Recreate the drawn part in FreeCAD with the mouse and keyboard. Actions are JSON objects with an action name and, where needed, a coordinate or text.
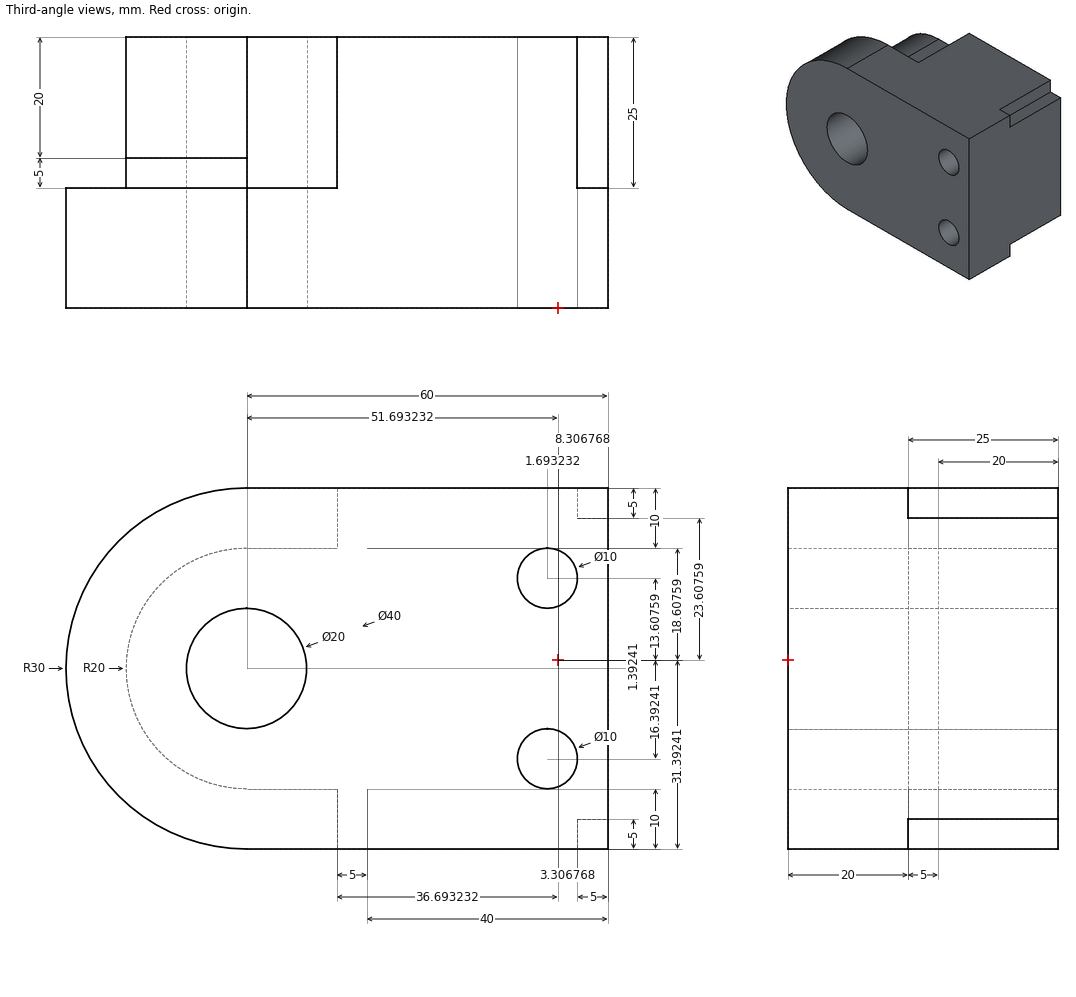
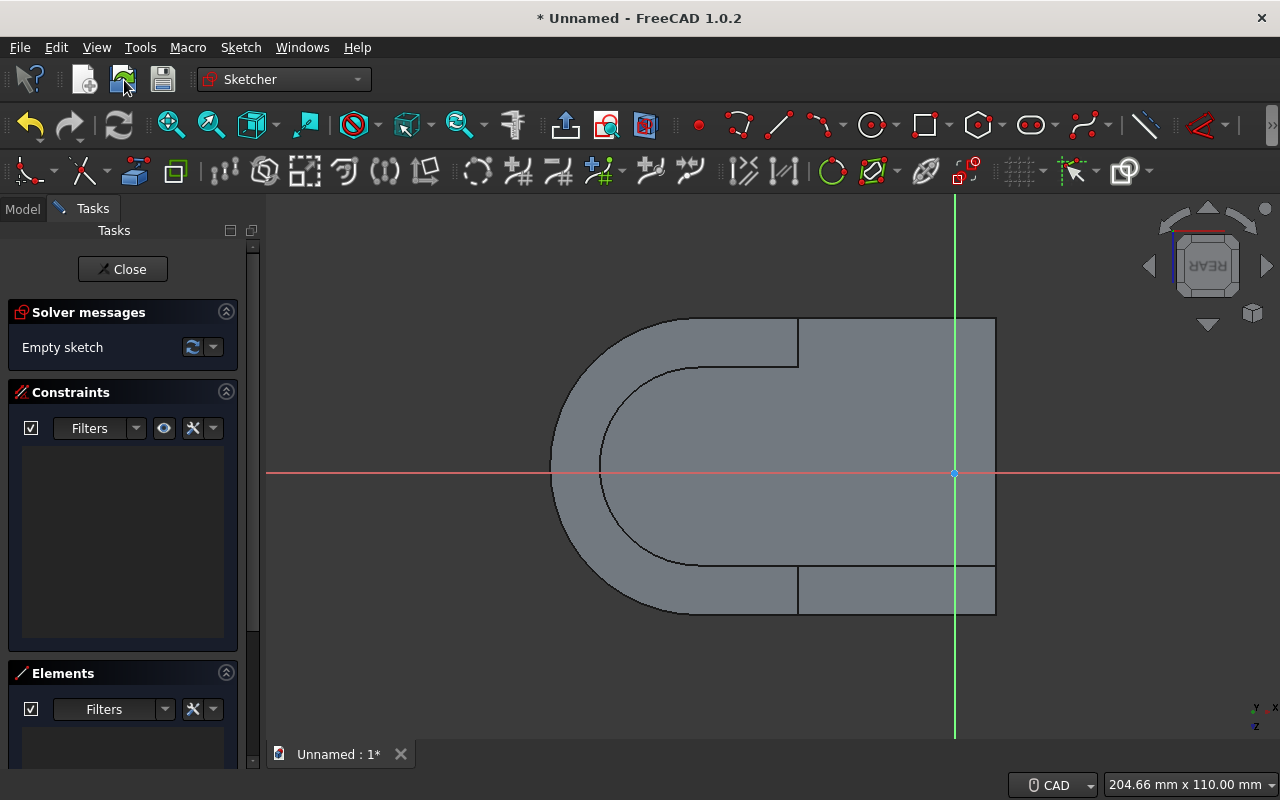
{"action": "scroll", "coordinate": [1054, 608], "scroll_direction": "up", "scroll_amount": 4}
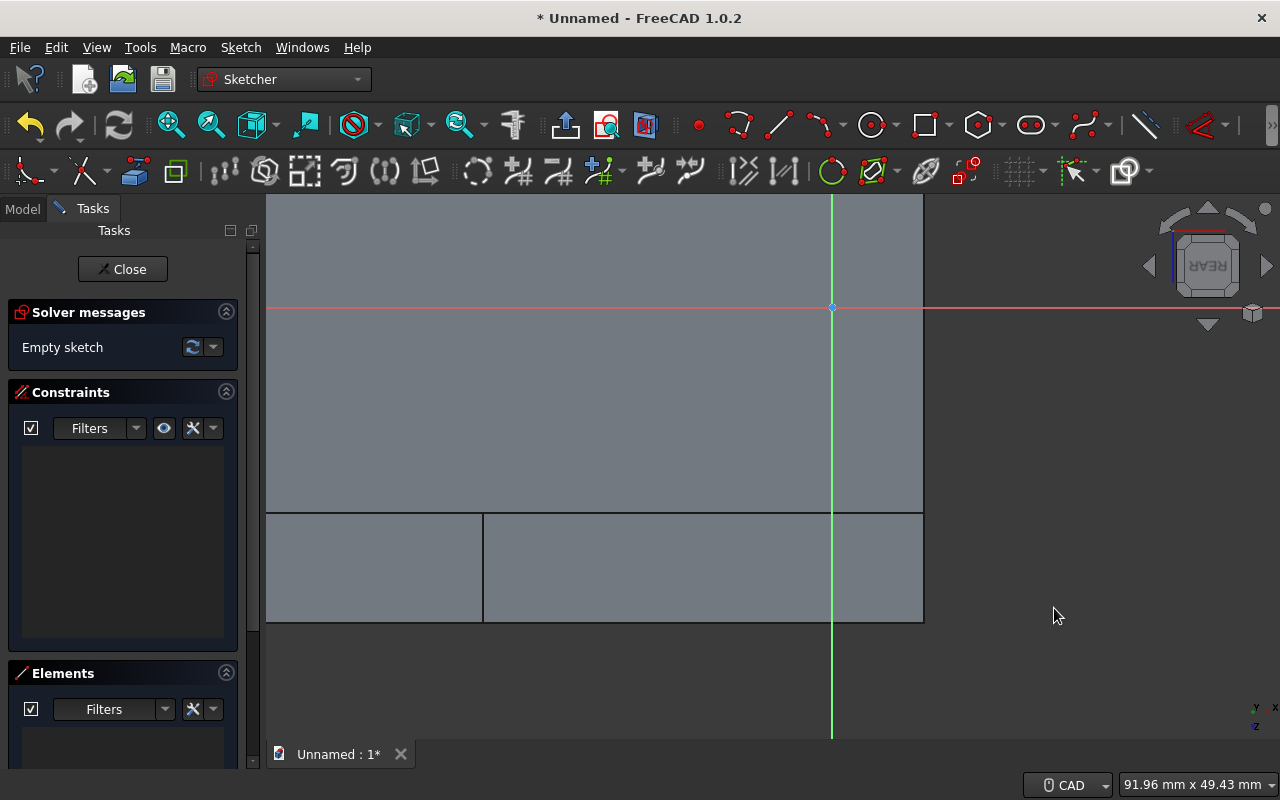
{"action": "left_click", "coordinate": [926, 126]}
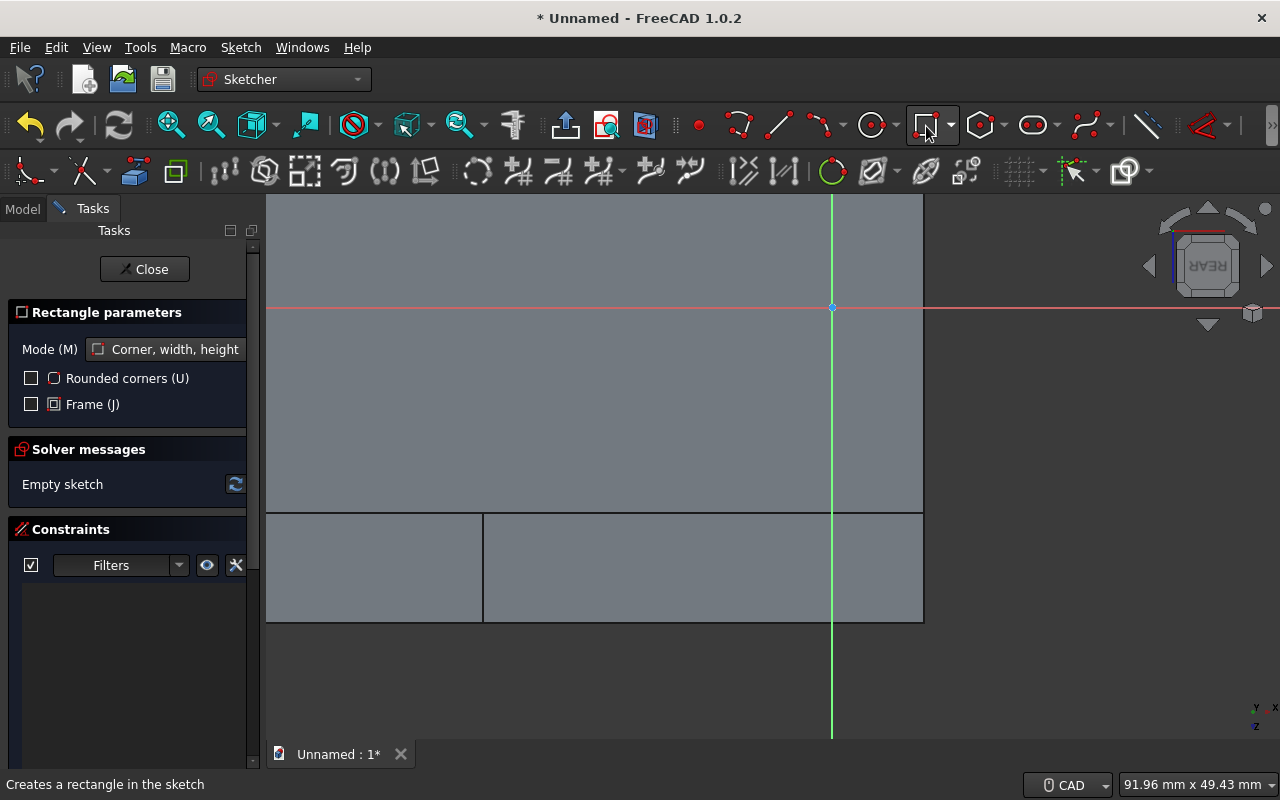
{"action": "left_click", "coordinate": [483, 513]}
{"action": "left_click", "coordinate": [924, 623]}
{"action": "key", "text": "Escape"}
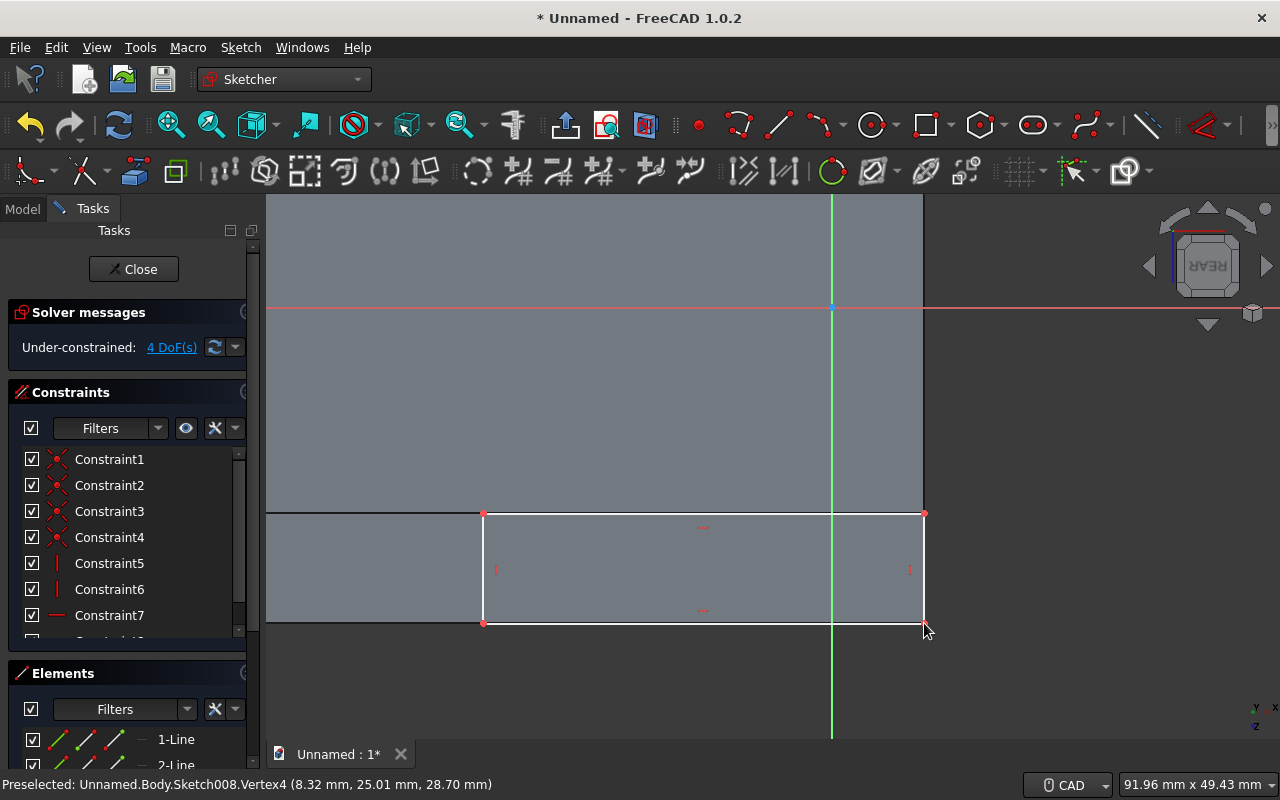
{"action": "key", "text": "d"}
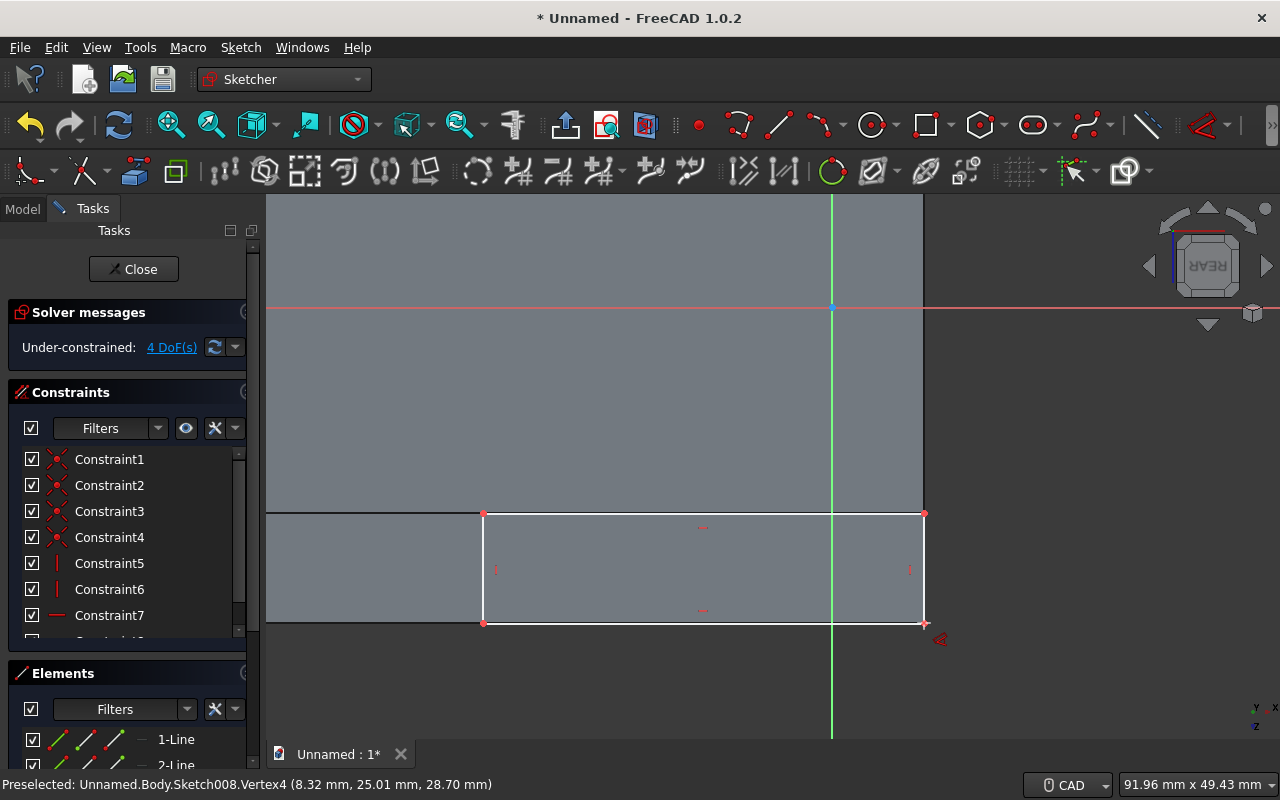
{"action": "left_click", "coordinate": [483, 547]}
{"action": "left_click", "coordinate": [449, 569]}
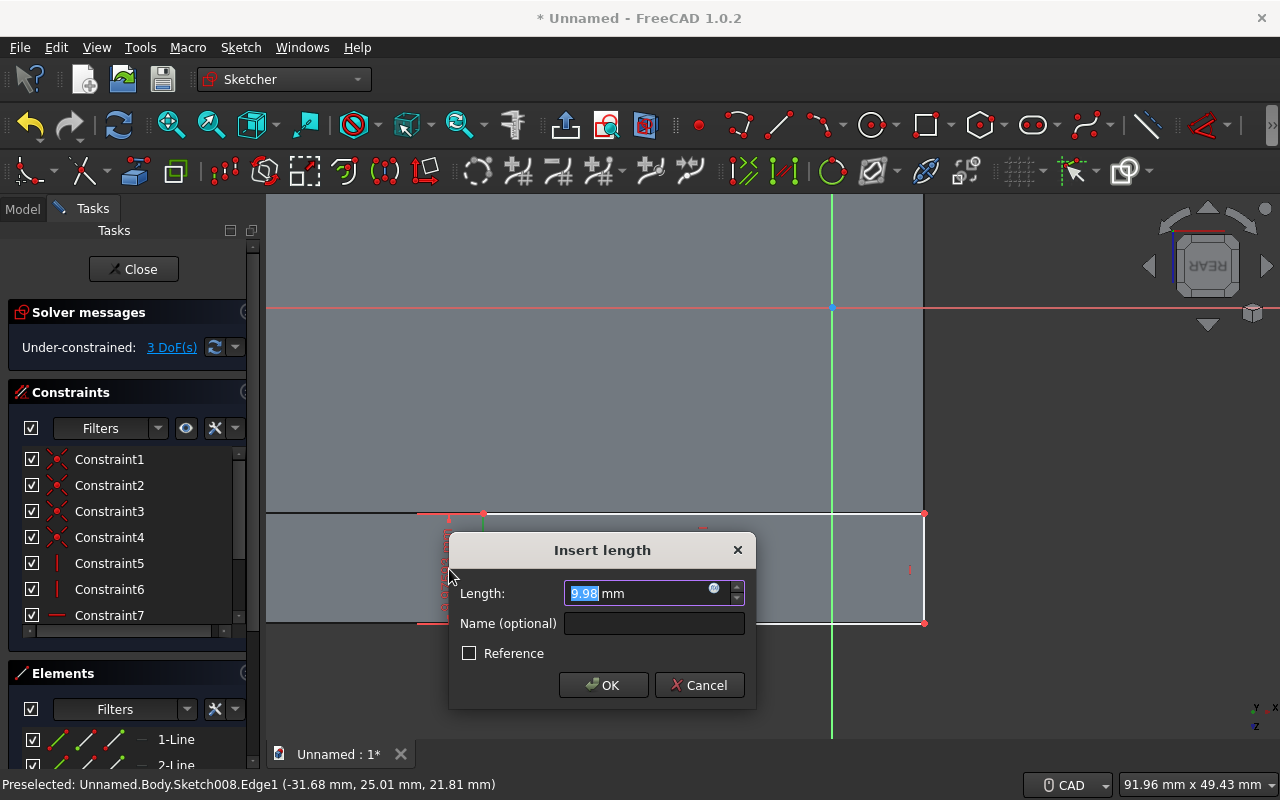
{"action": "type", "text": "10"}
{"action": "key", "text": "Return"}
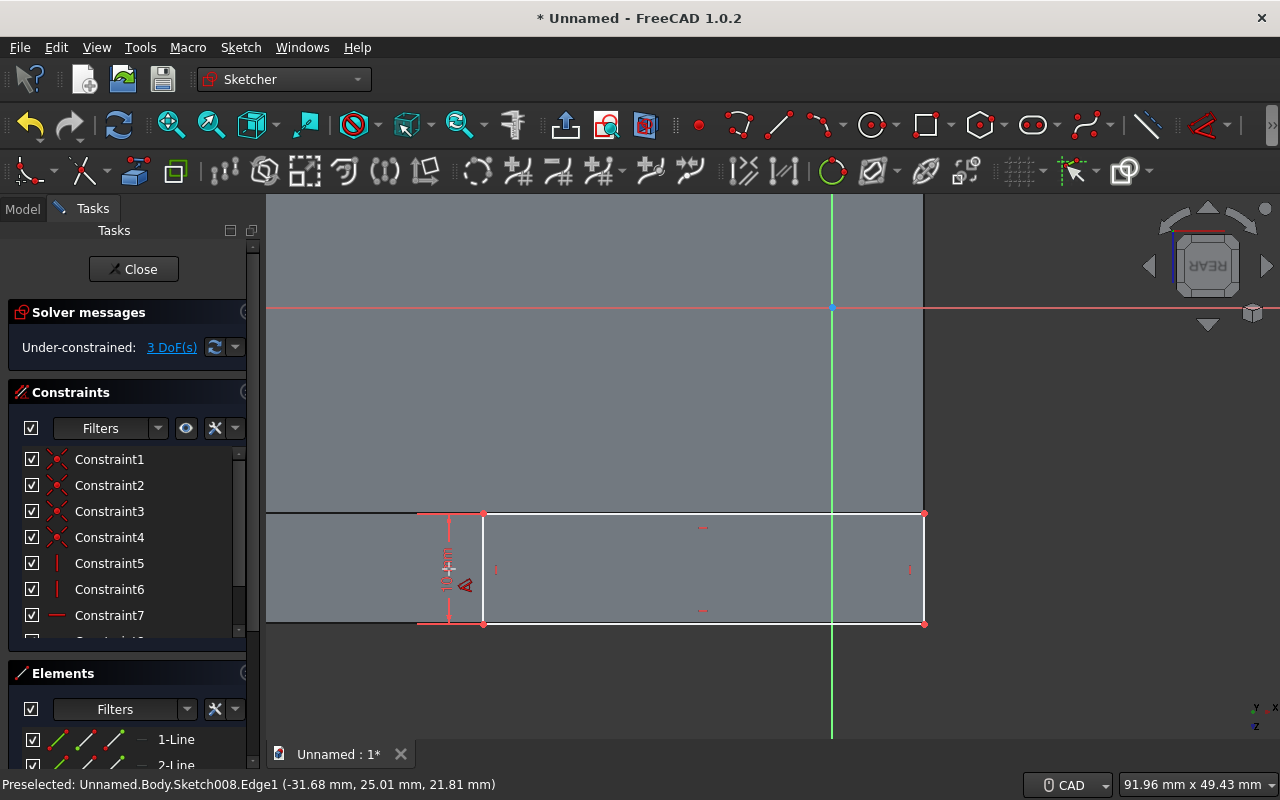
{"action": "left_click", "coordinate": [615, 624]}
{"action": "left_click", "coordinate": [703, 658]}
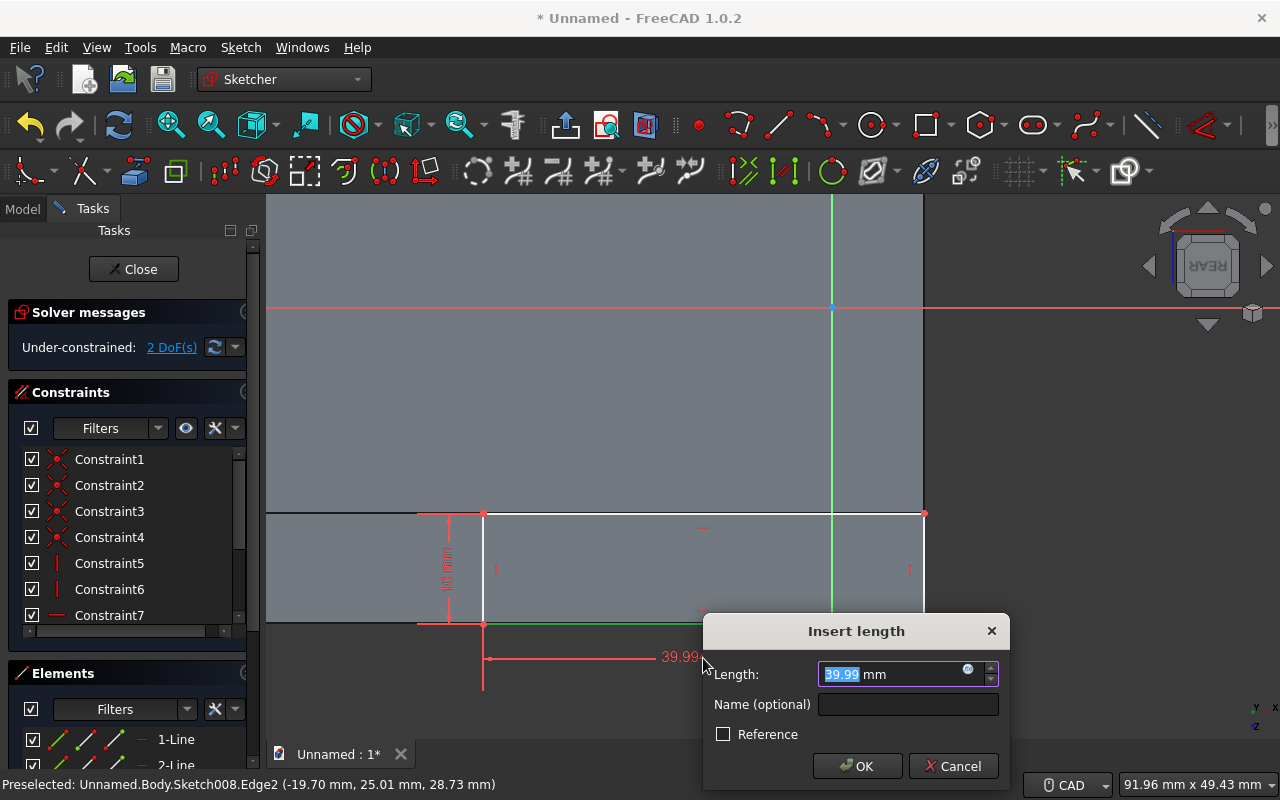
{"action": "type", "text": "40"}
{"action": "key", "text": "Return"}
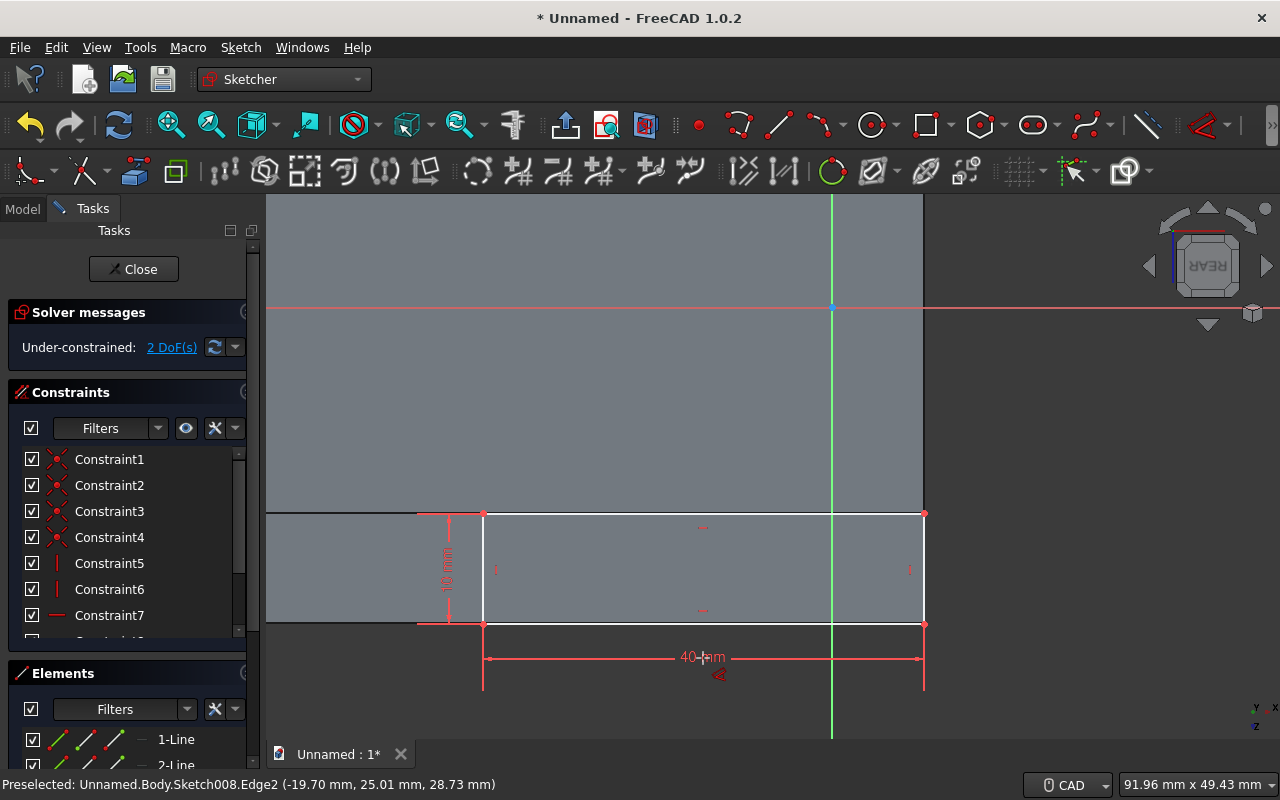
{"action": "left_click", "coordinate": [483, 514]}
{"action": "left_click", "coordinate": [449, 411]}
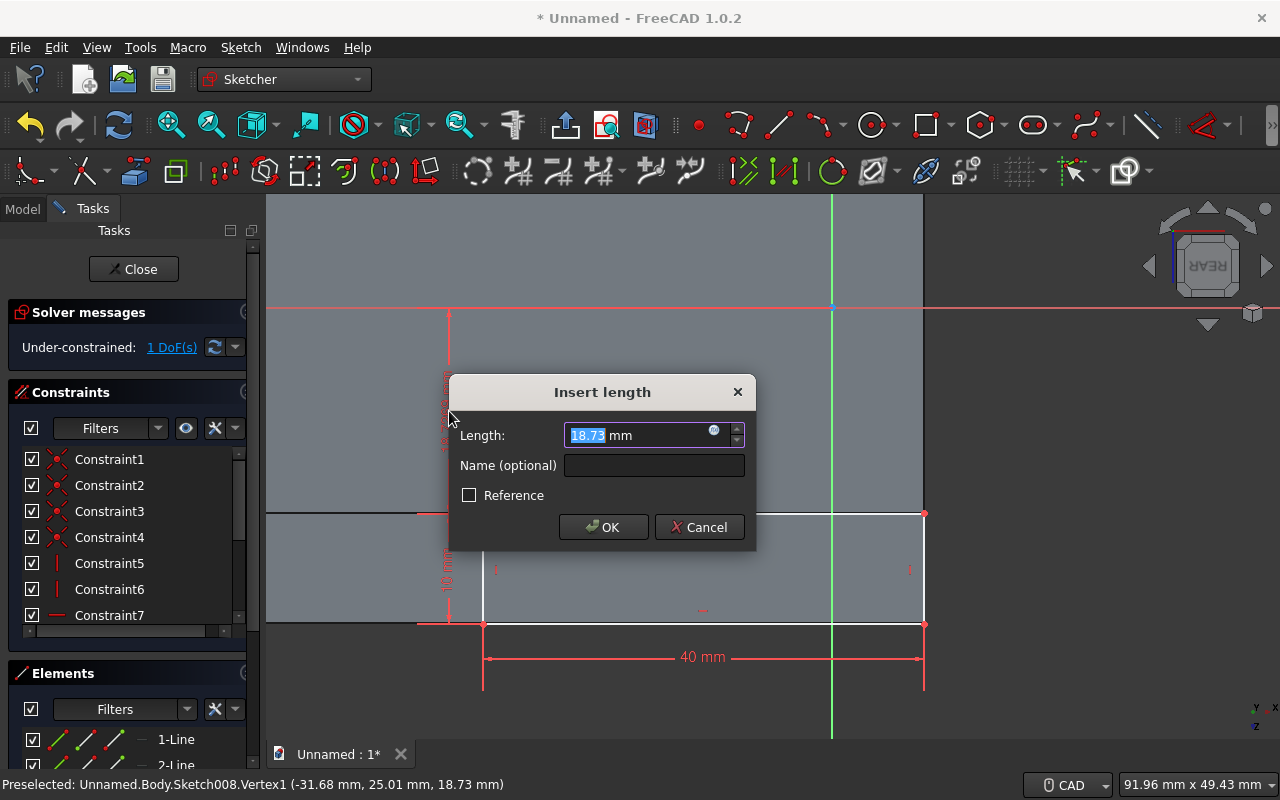
{"action": "type", "text": "18.60759"}
{"action": "key", "text": "Return"}